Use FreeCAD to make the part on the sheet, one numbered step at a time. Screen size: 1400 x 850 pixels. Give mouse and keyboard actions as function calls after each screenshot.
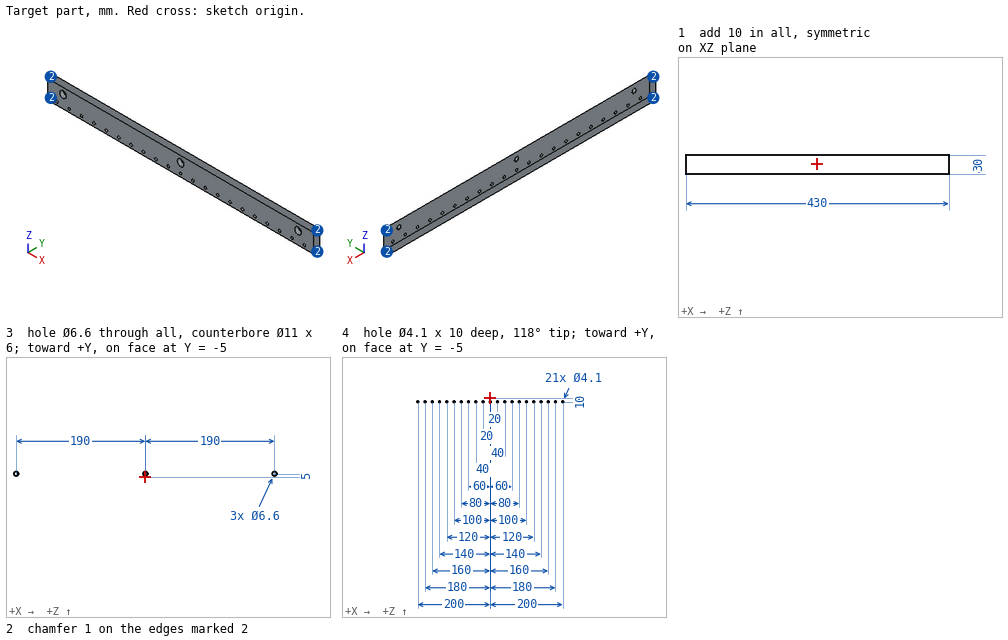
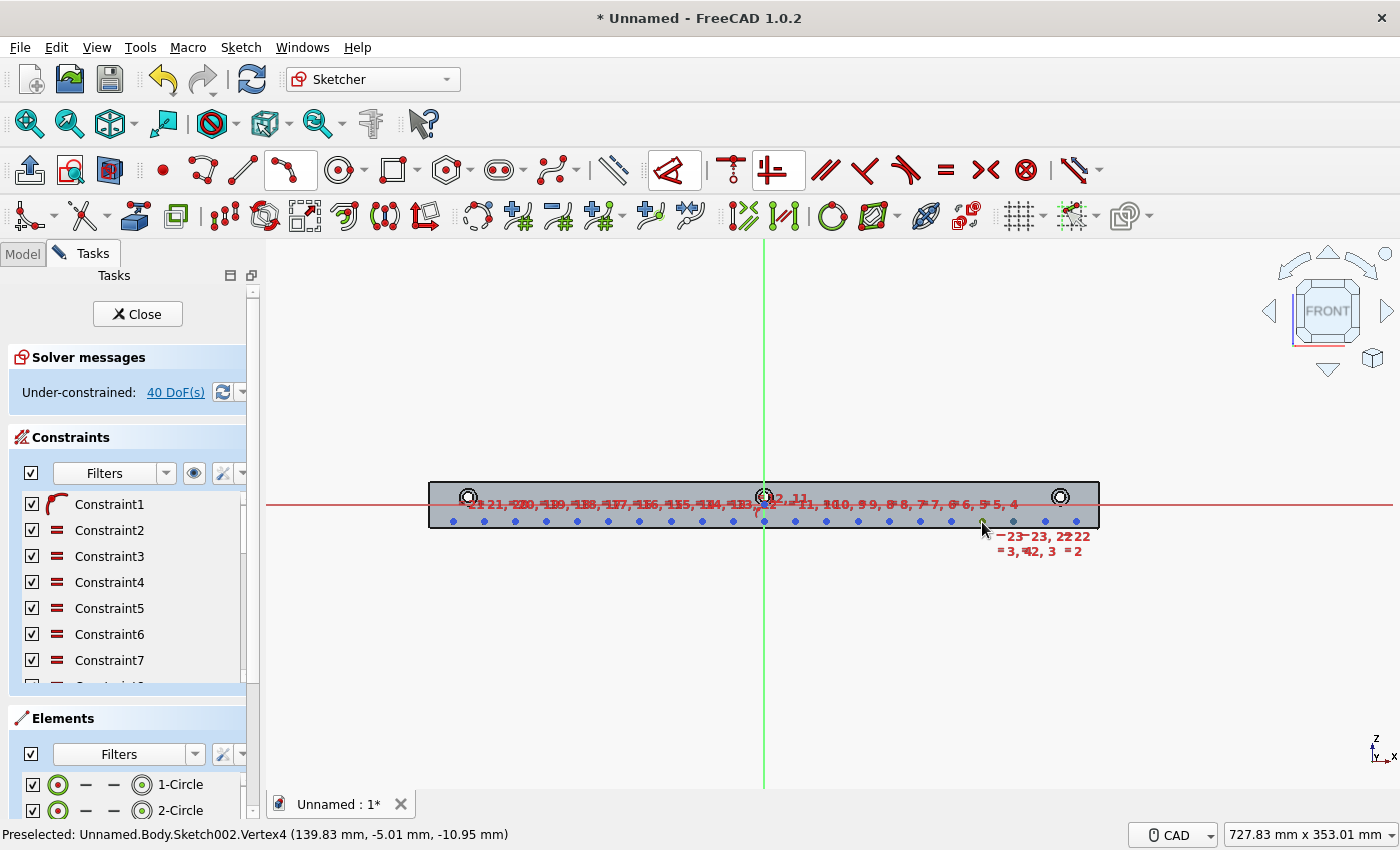
click(800, 170)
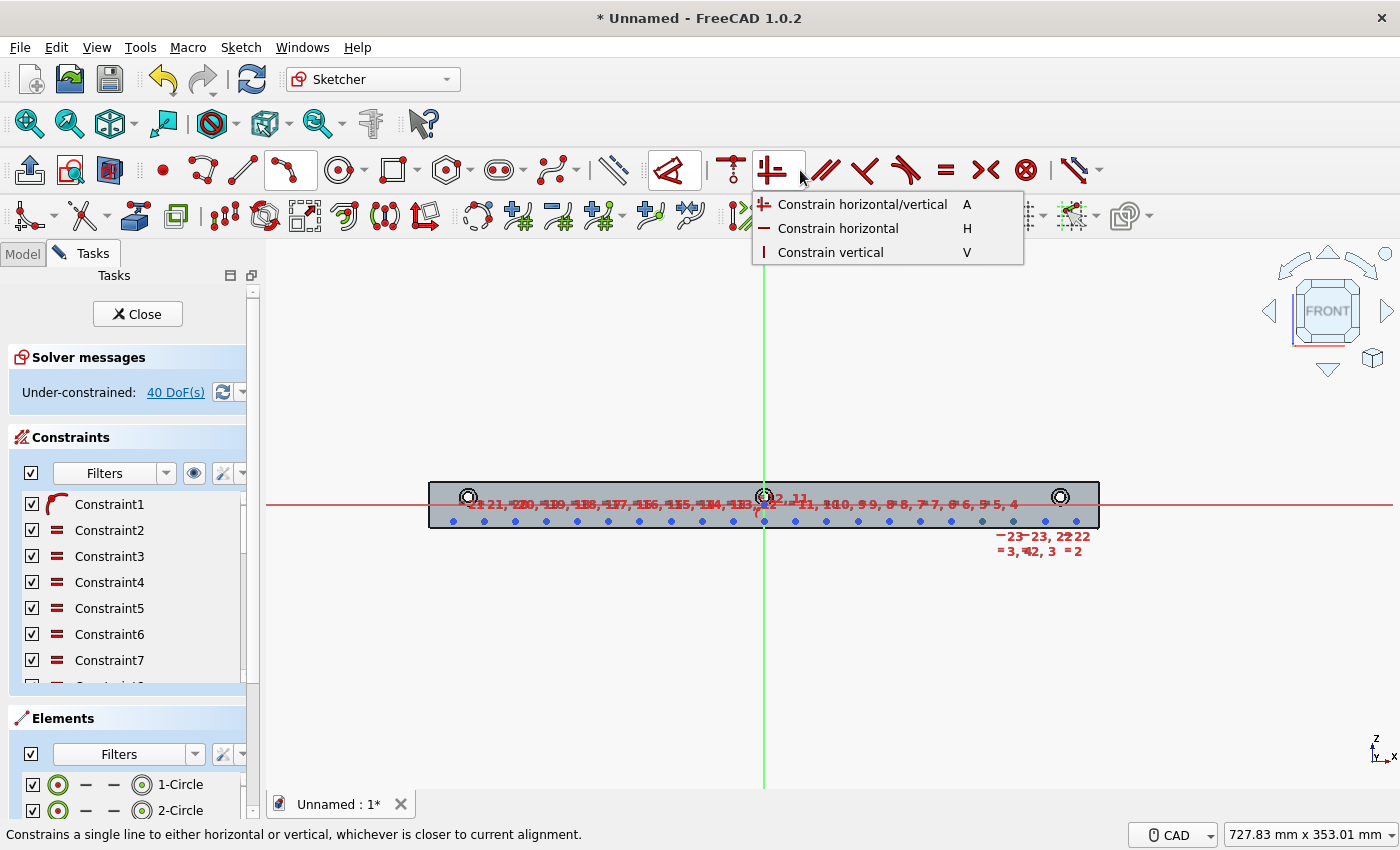
click(888, 228)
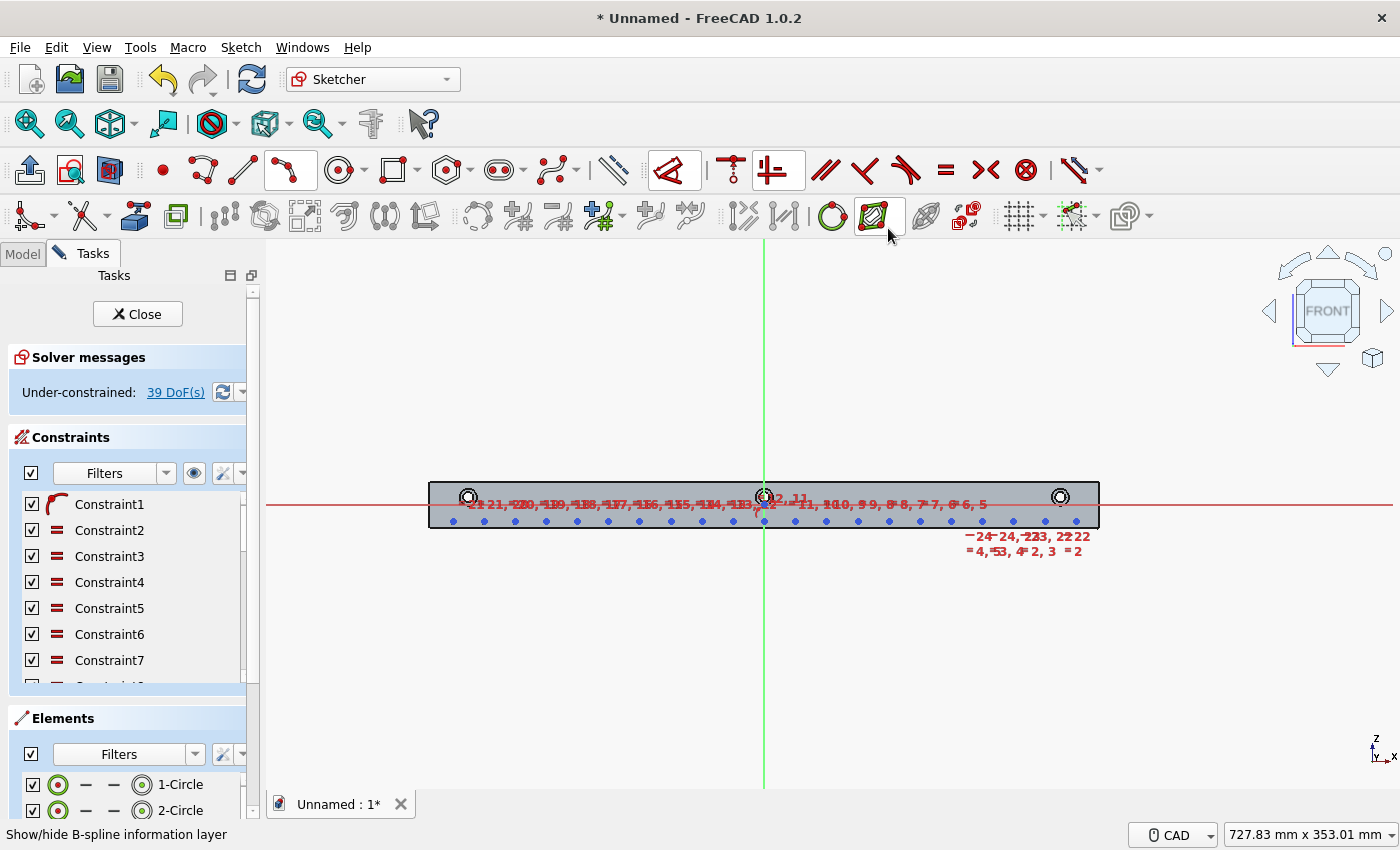
click(982, 522)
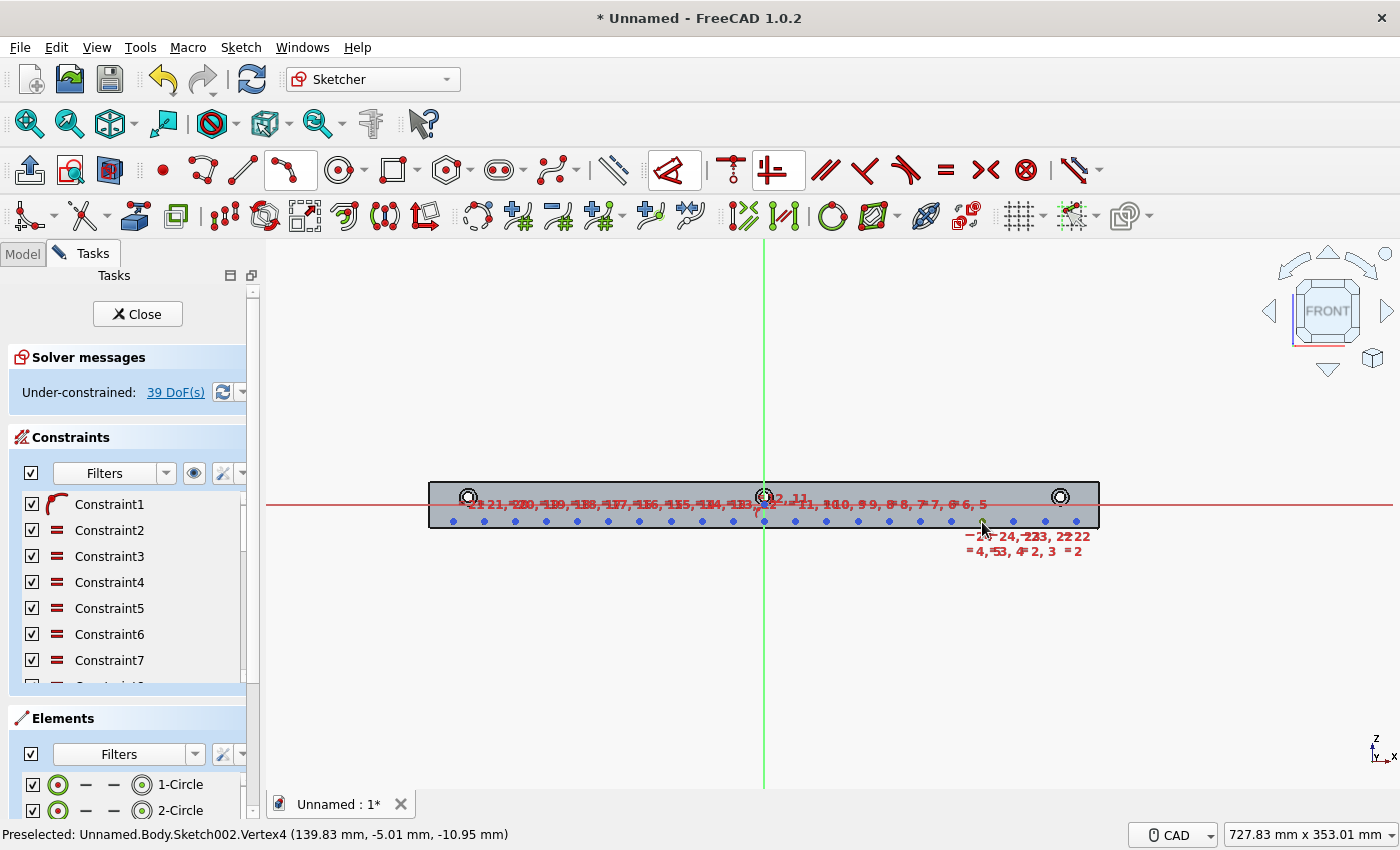
click(951, 522)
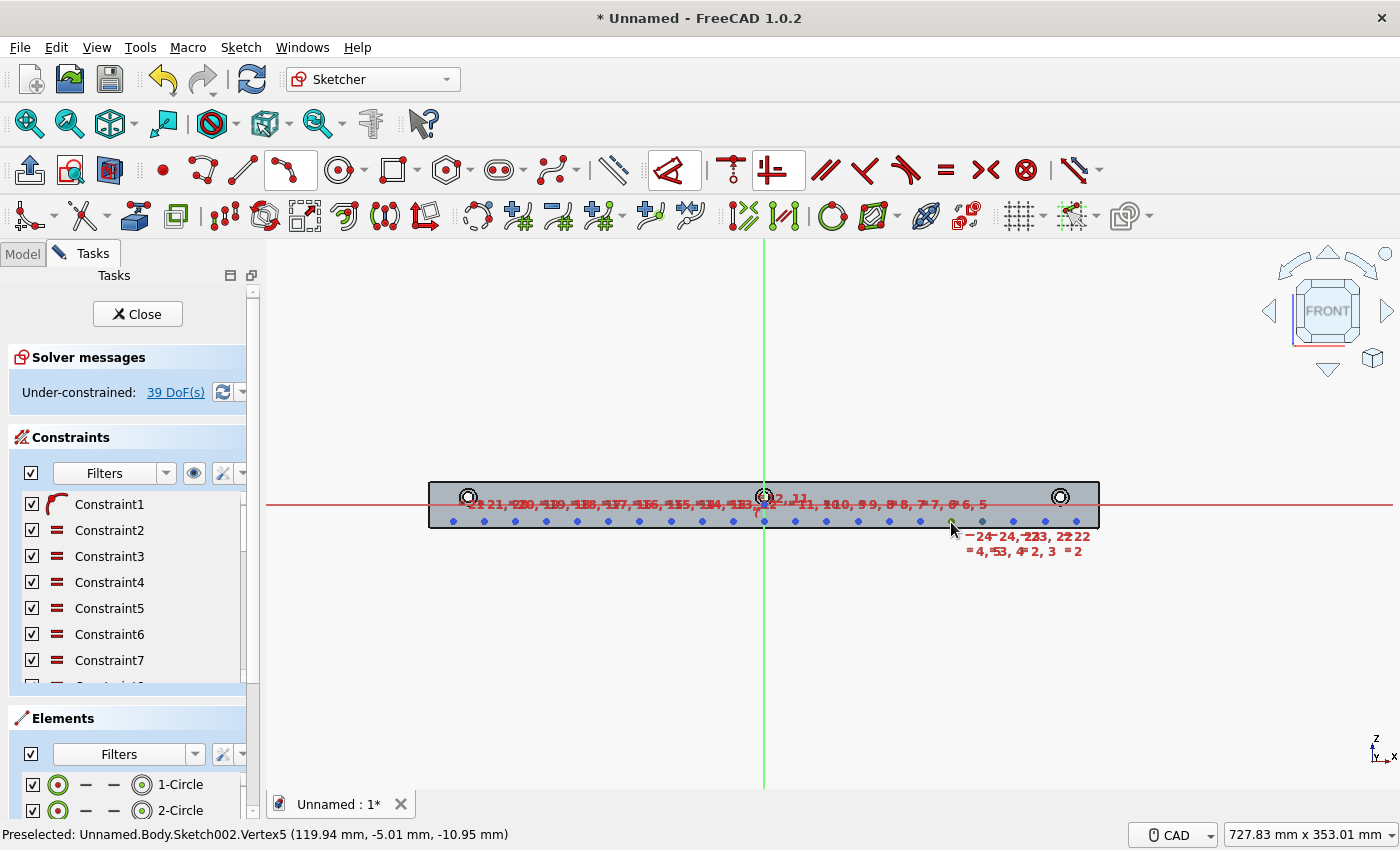
key(h)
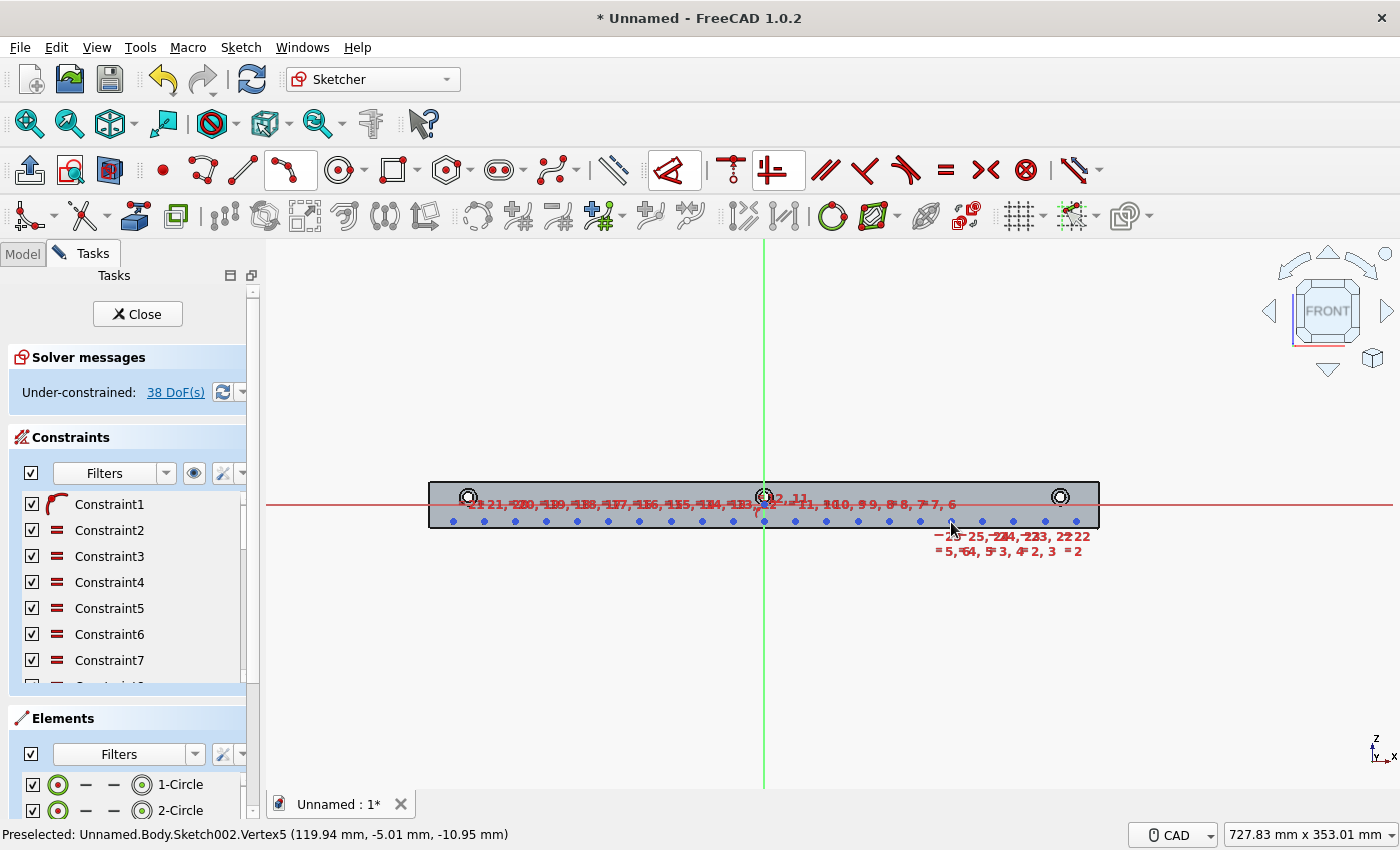
click(951, 522)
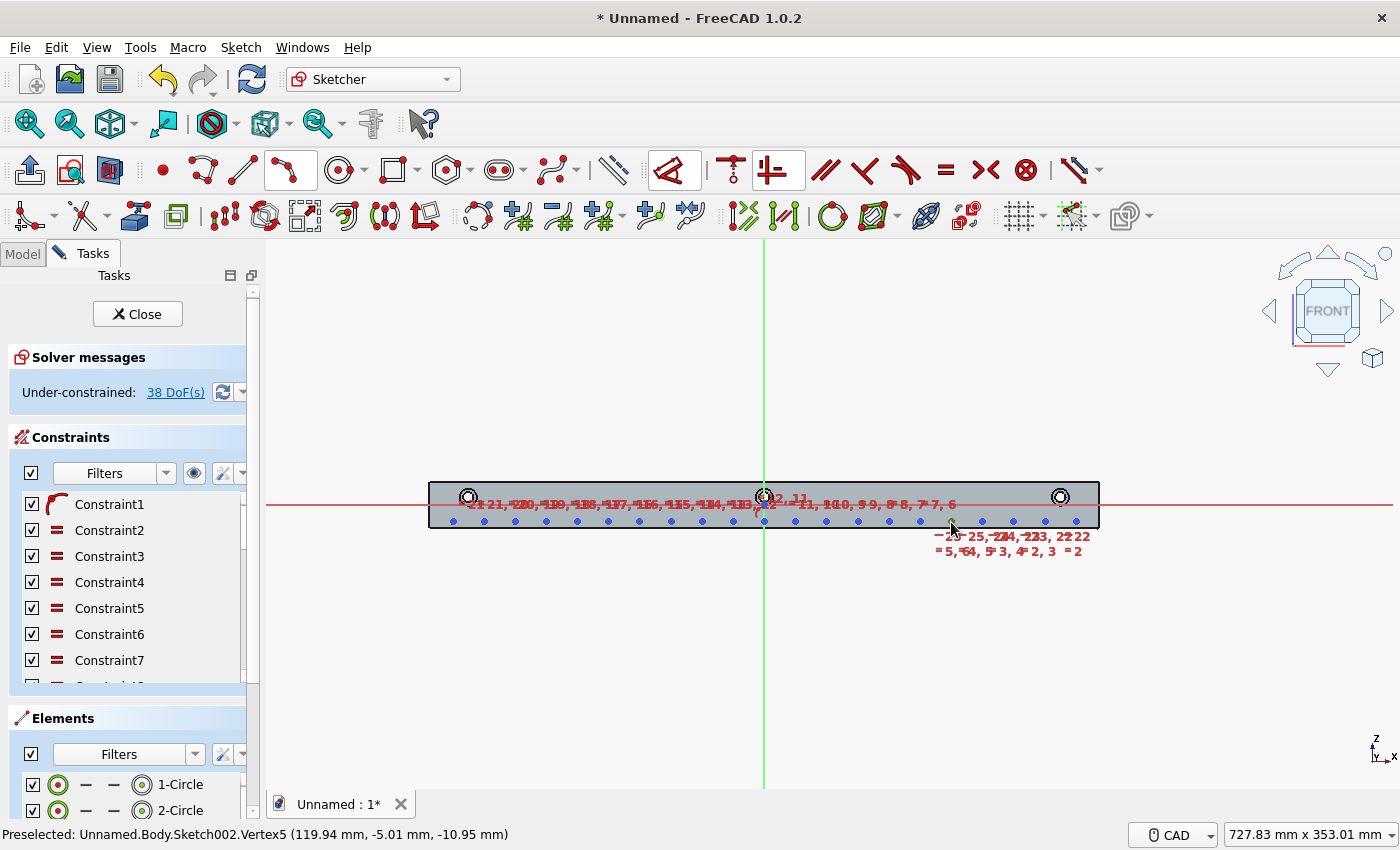
click(920, 522)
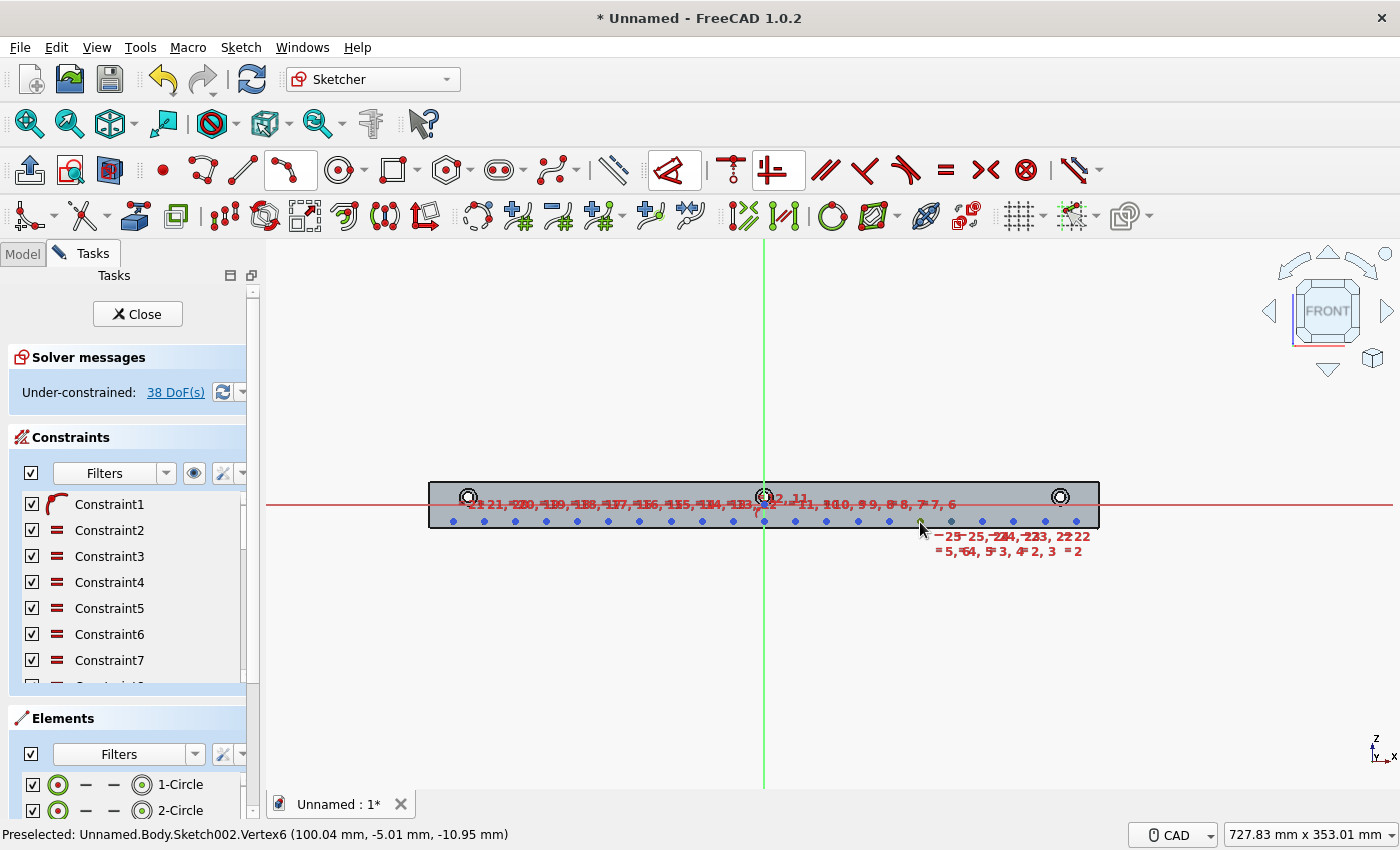
key(h)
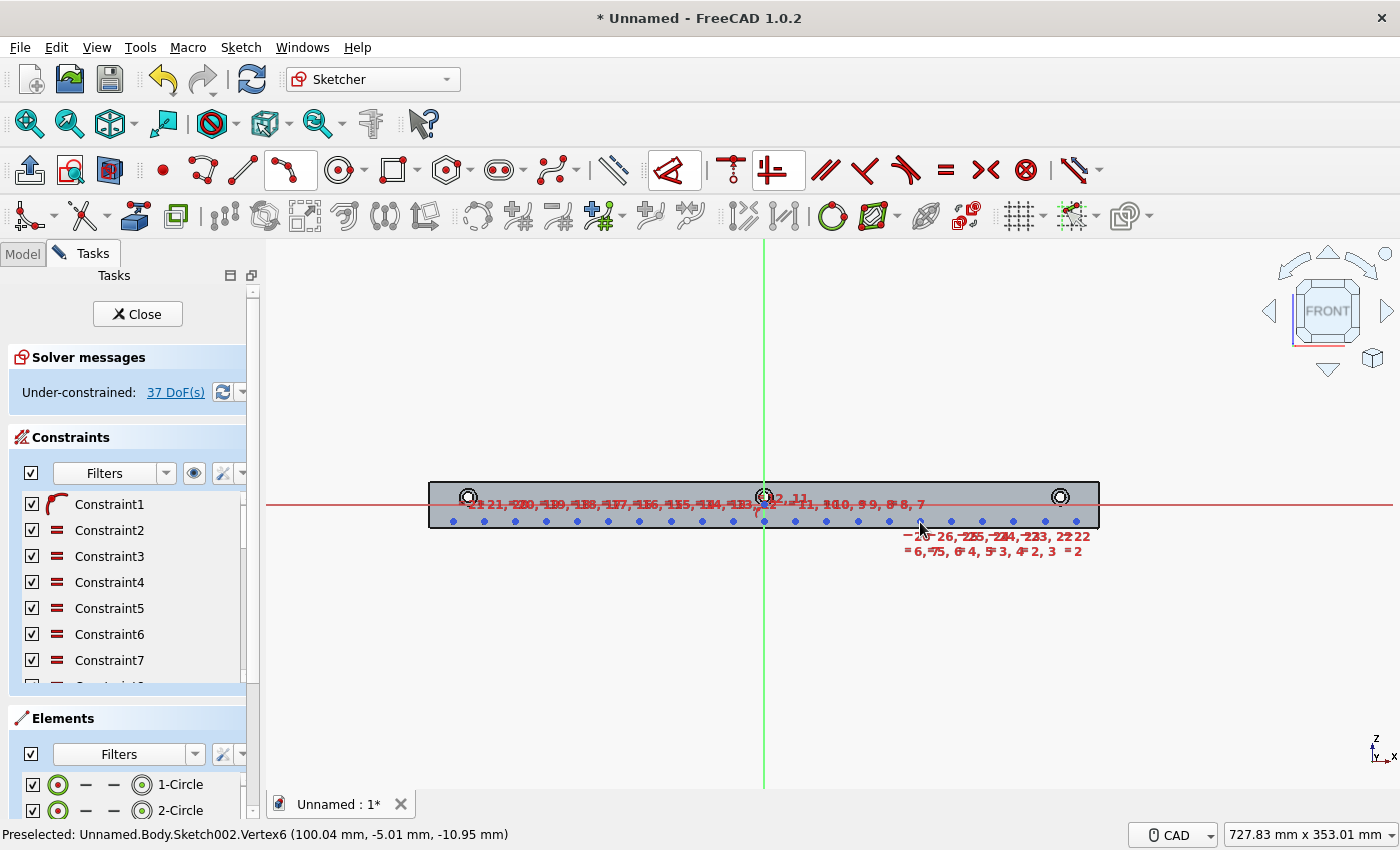
click(920, 522)